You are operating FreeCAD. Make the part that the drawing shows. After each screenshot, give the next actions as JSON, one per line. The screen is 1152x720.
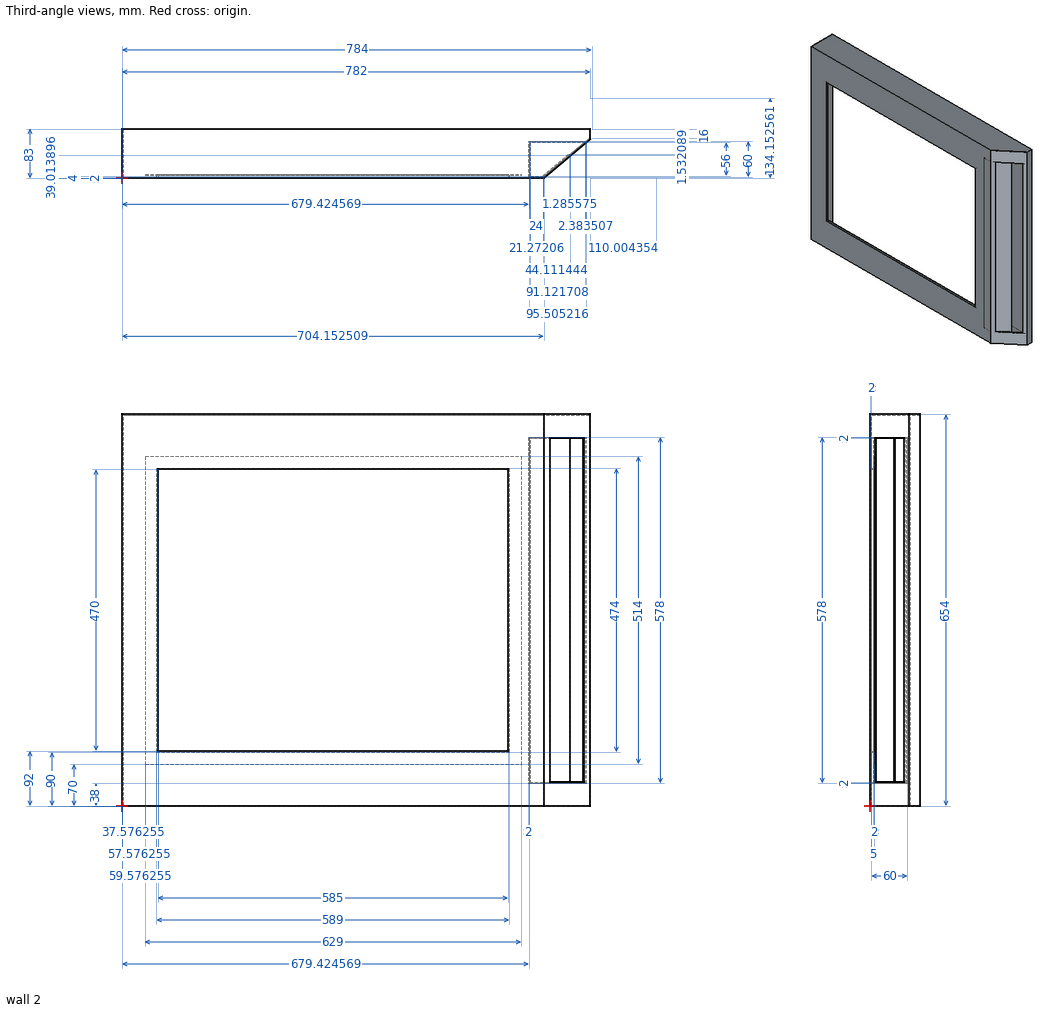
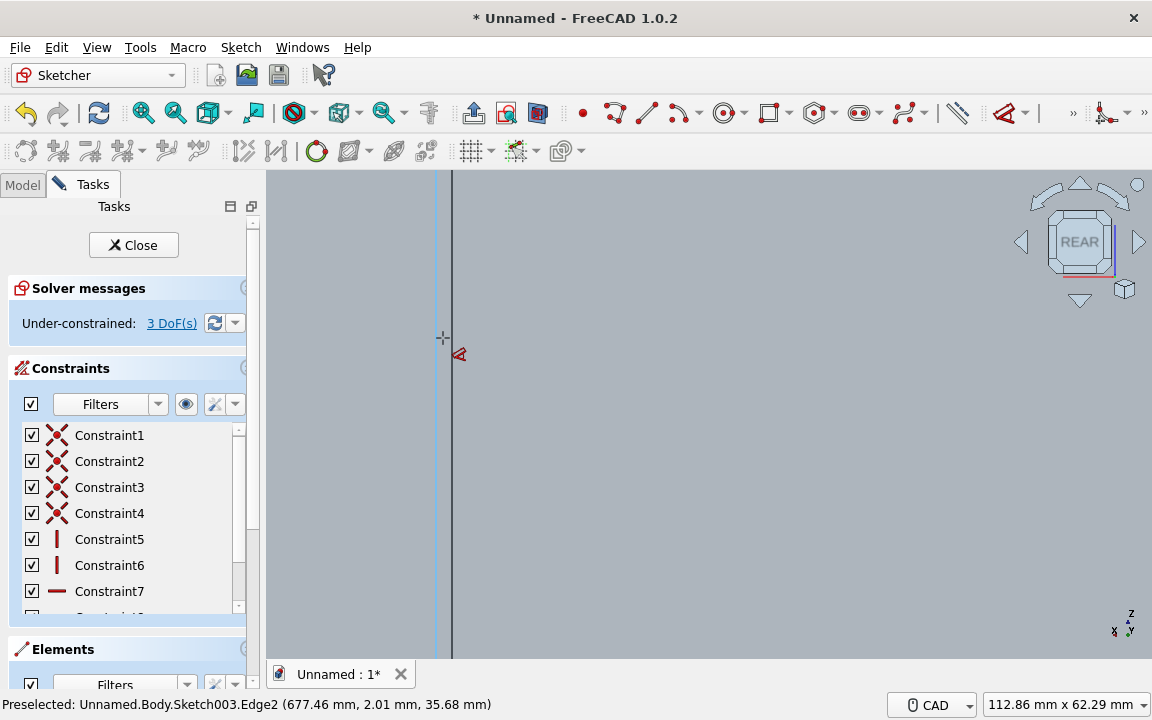
{"action": "left_click", "coordinate": [436, 335]}
{"action": "left_click", "coordinate": [402, 414]}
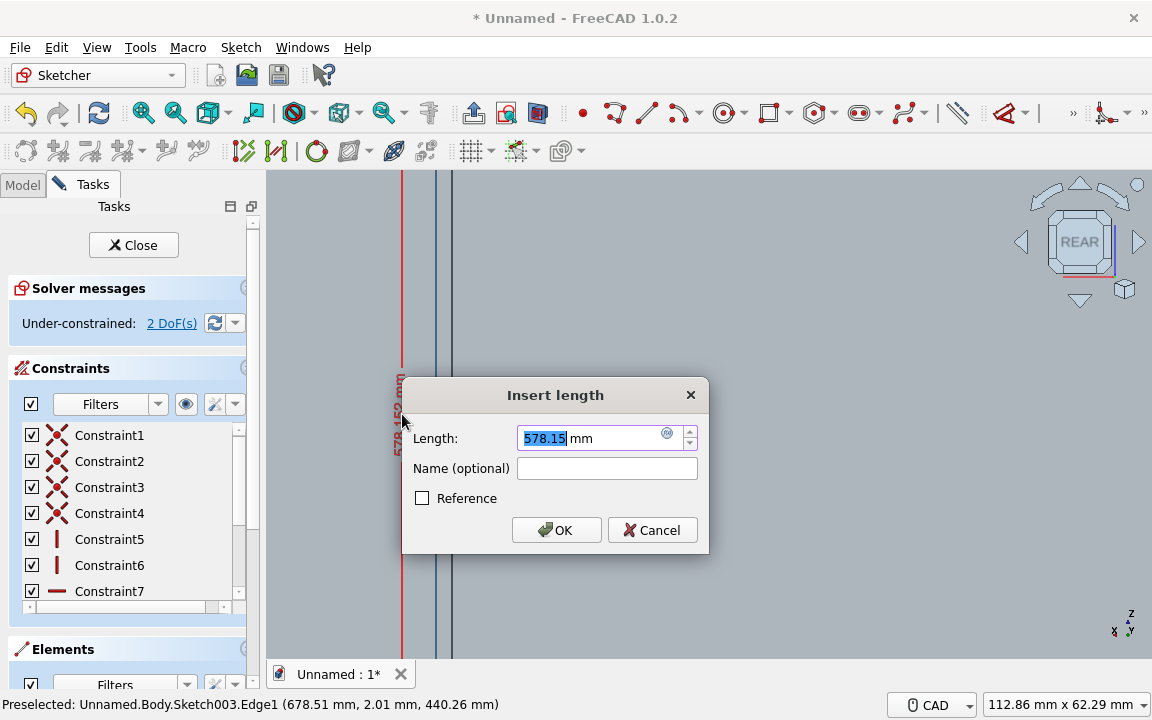
{"action": "type", "text": "578"}
{"action": "key", "text": "Return"}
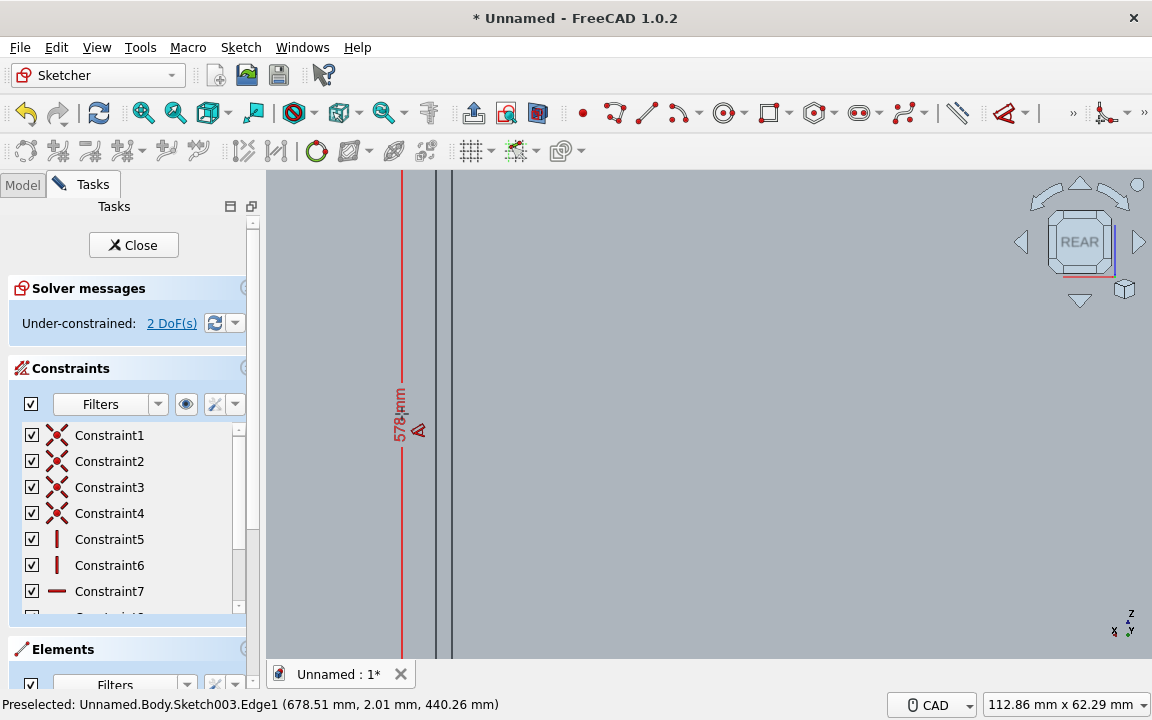
{"action": "scroll", "coordinate": [482, 352], "scroll_direction": "down", "scroll_amount": 14}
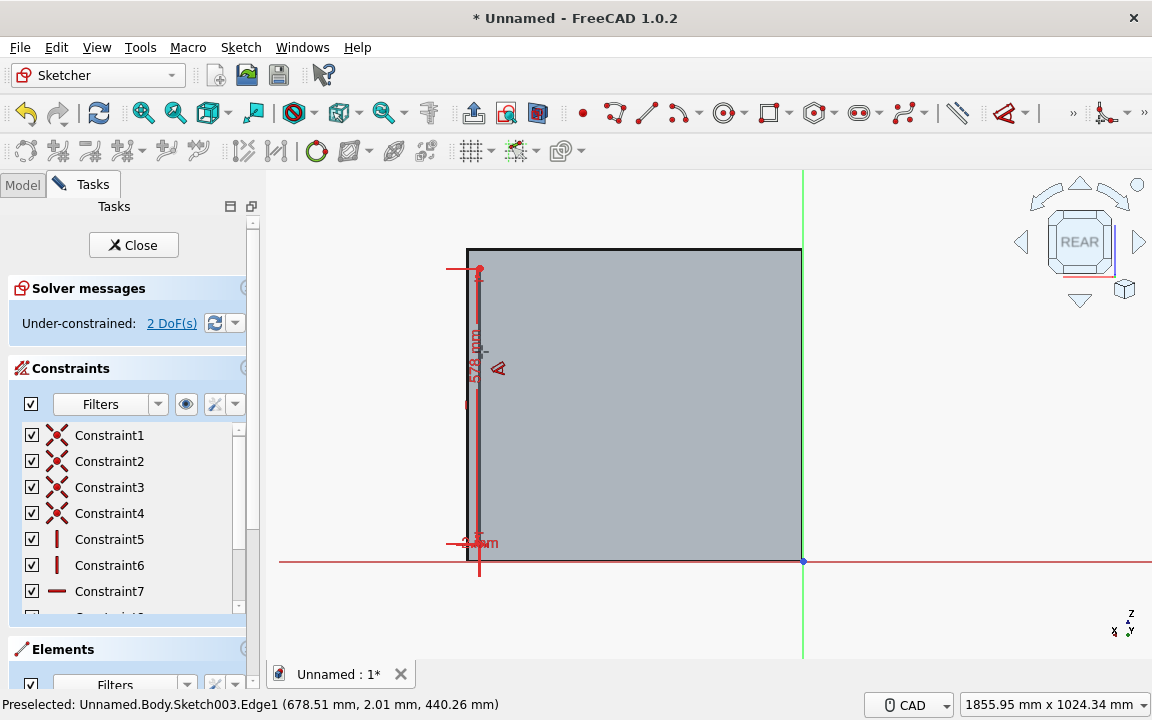
{"action": "scroll", "coordinate": [479, 544], "scroll_direction": "up", "scroll_amount": 13}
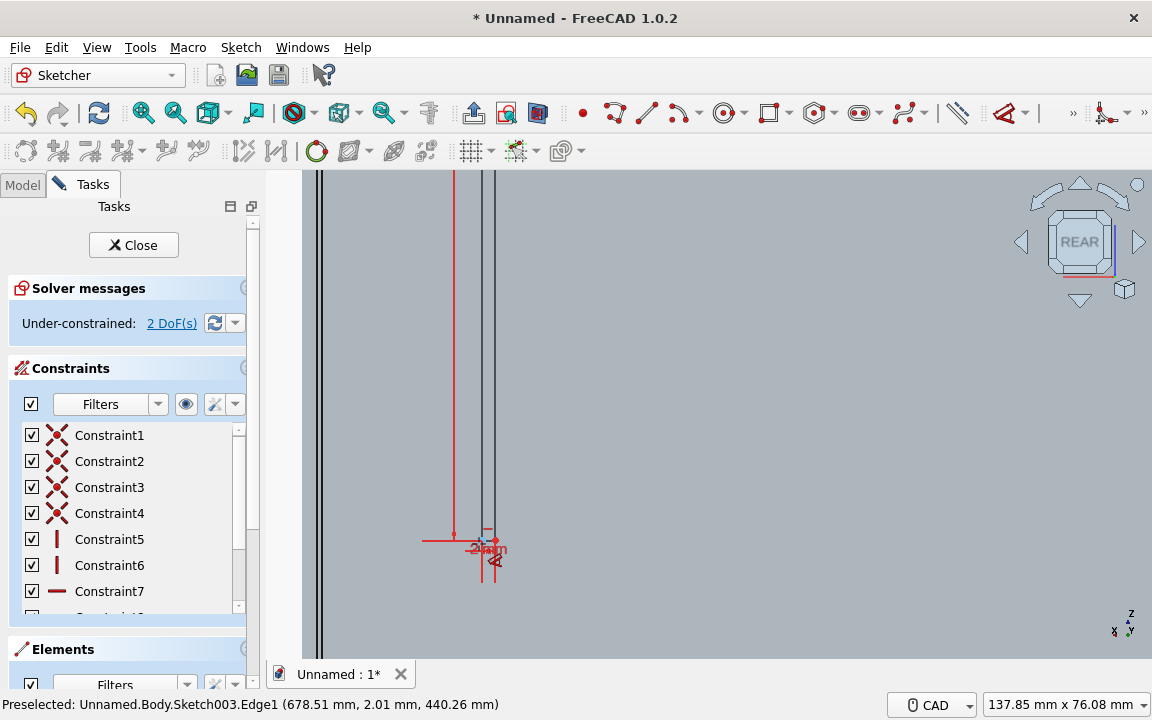
{"action": "left_click", "coordinate": [482, 541]}
{"action": "left_click", "coordinate": [448, 586]}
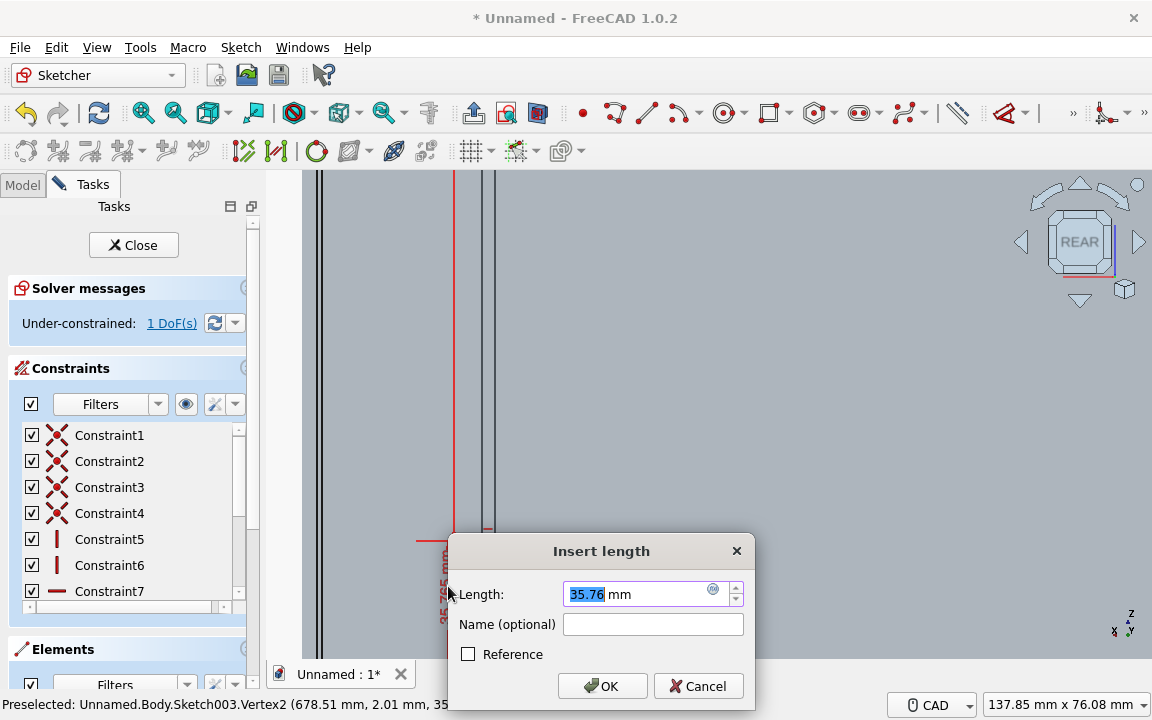
{"action": "type", "text": "38"}
{"action": "key", "text": "Return"}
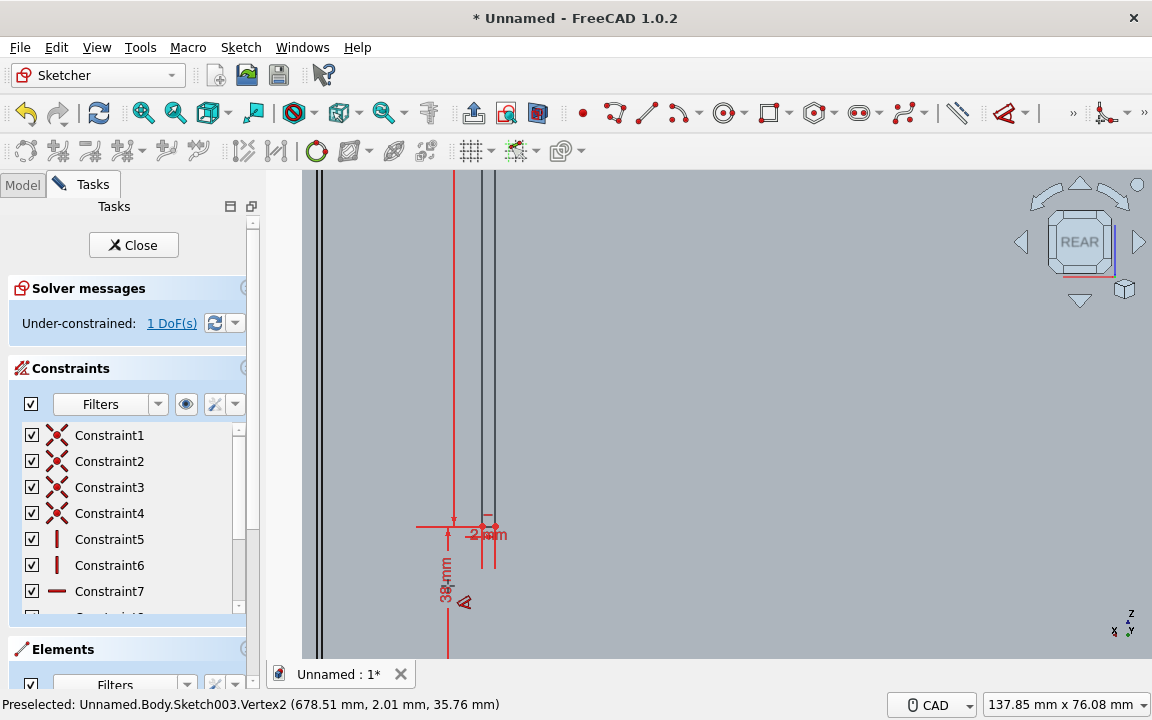
{"action": "scroll", "coordinate": [478, 545], "scroll_direction": "down", "scroll_amount": 13}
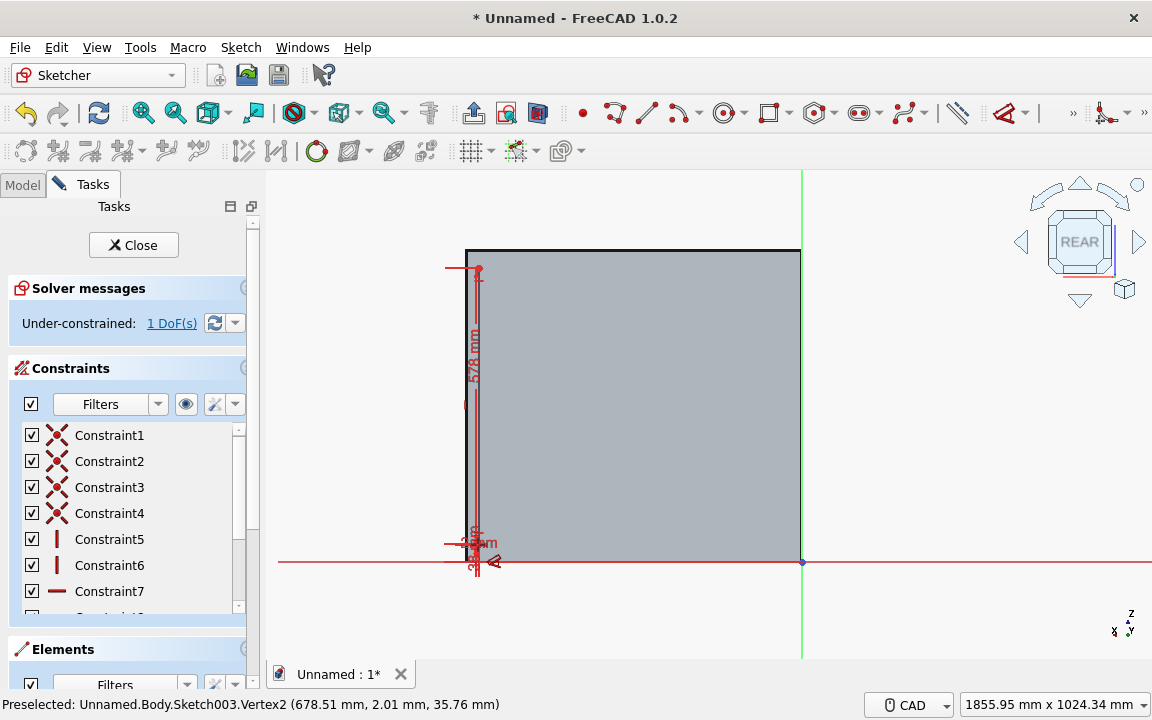
{"action": "scroll", "coordinate": [479, 268], "scroll_direction": "up", "scroll_amount": 13}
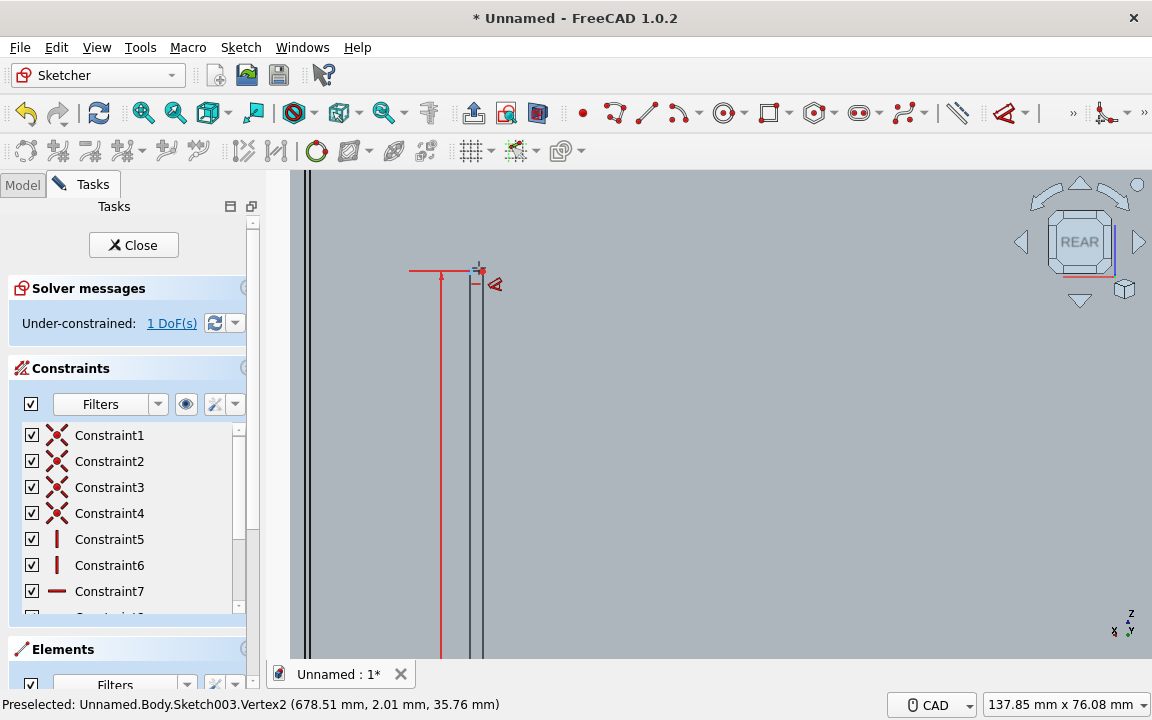
{"action": "left_click", "coordinate": [470, 271]}
{"action": "left_click", "coordinate": [728, 237]}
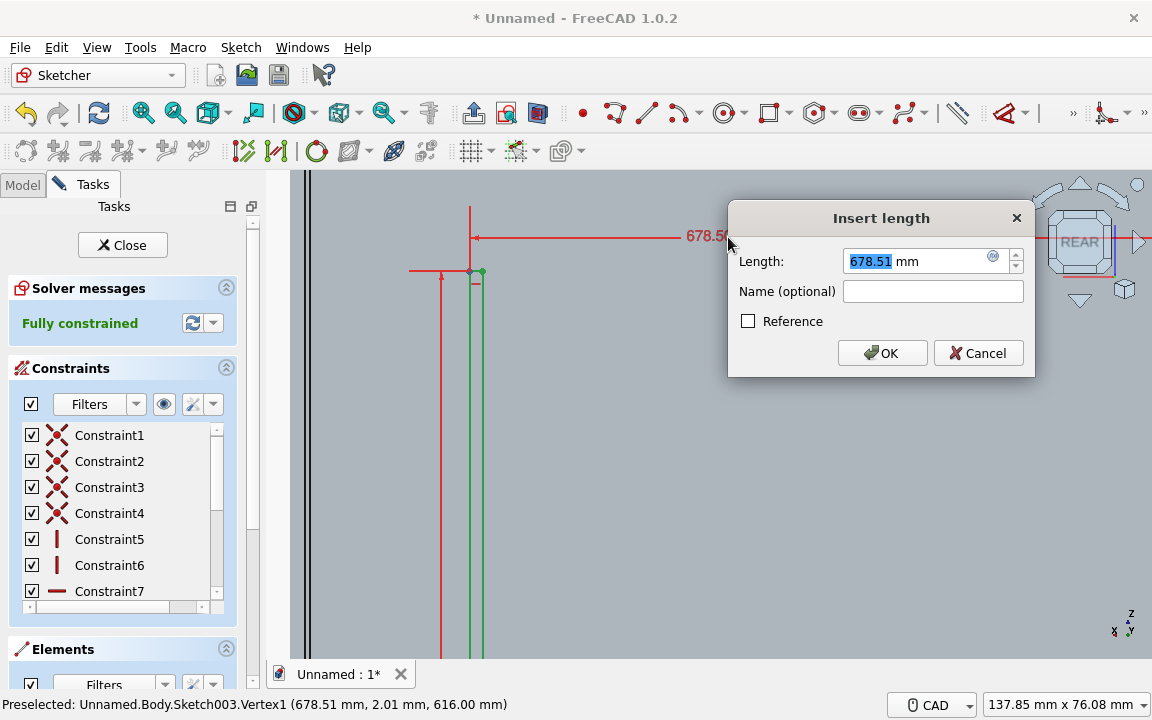
{"action": "type", "text": "679.424569"}
{"action": "key", "text": "Return"}
{"action": "key", "text": "Escape"}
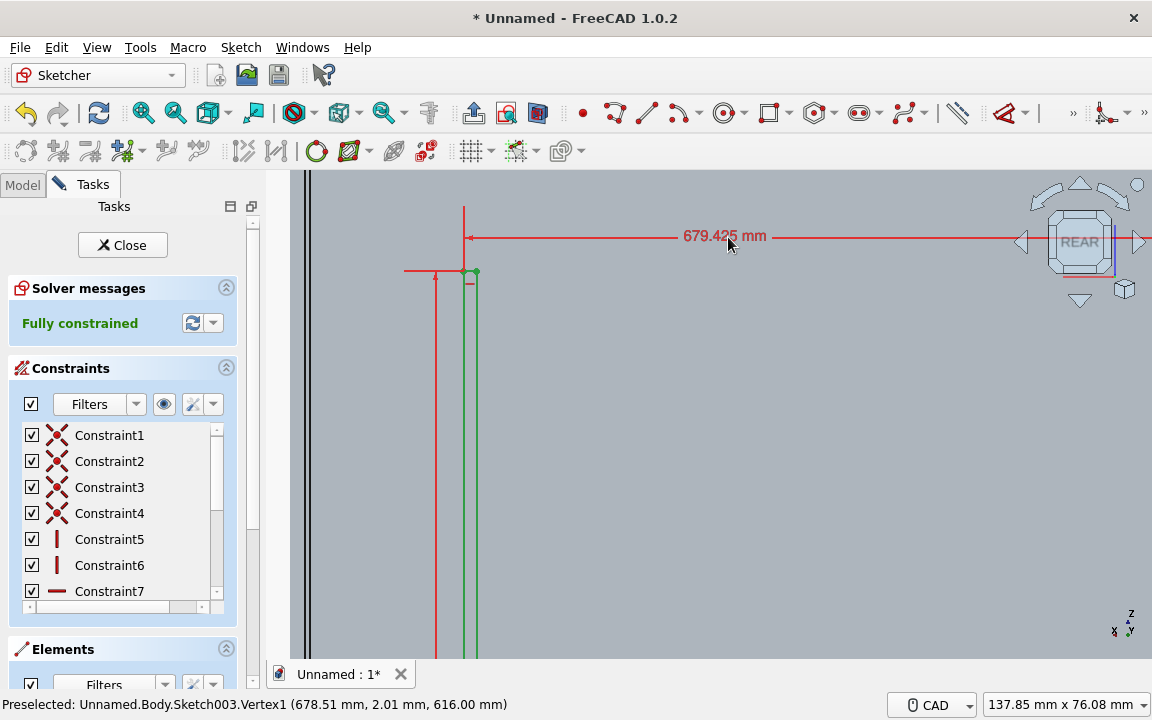
{"action": "left_click", "coordinate": [123, 245]}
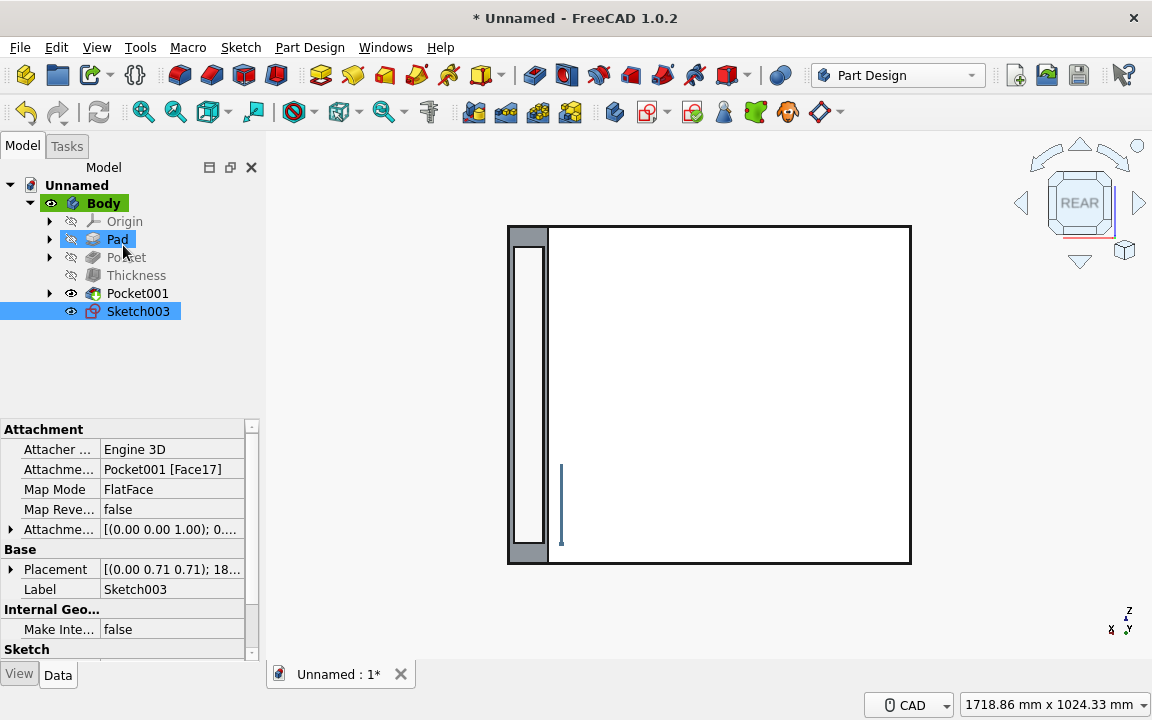
{"action": "left_click", "coordinate": [322, 76]}